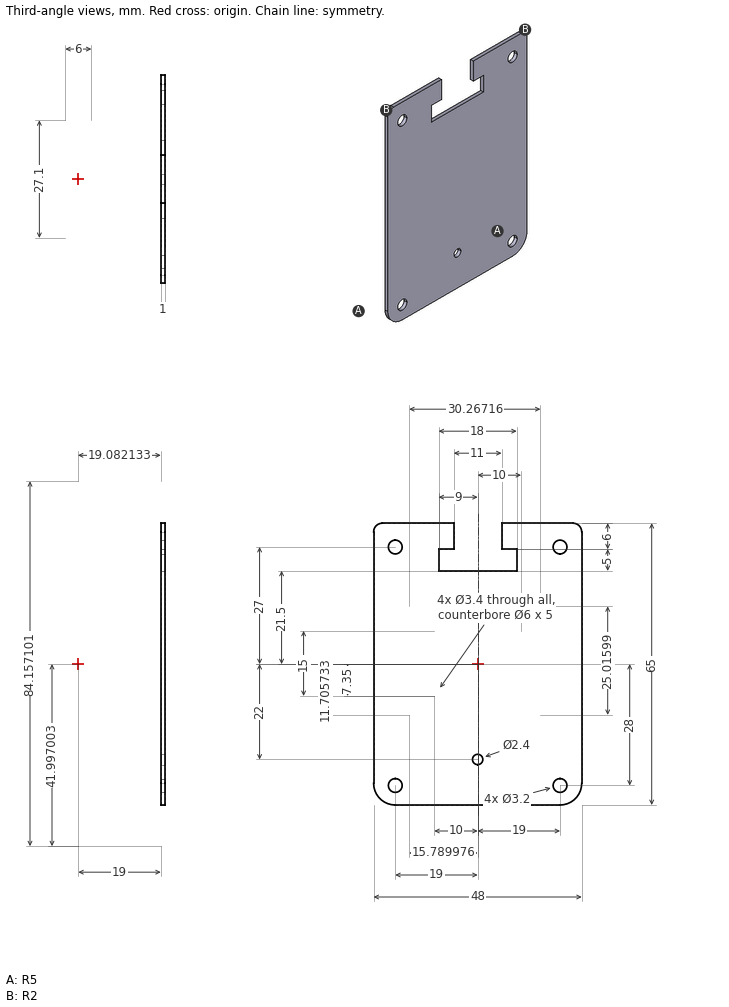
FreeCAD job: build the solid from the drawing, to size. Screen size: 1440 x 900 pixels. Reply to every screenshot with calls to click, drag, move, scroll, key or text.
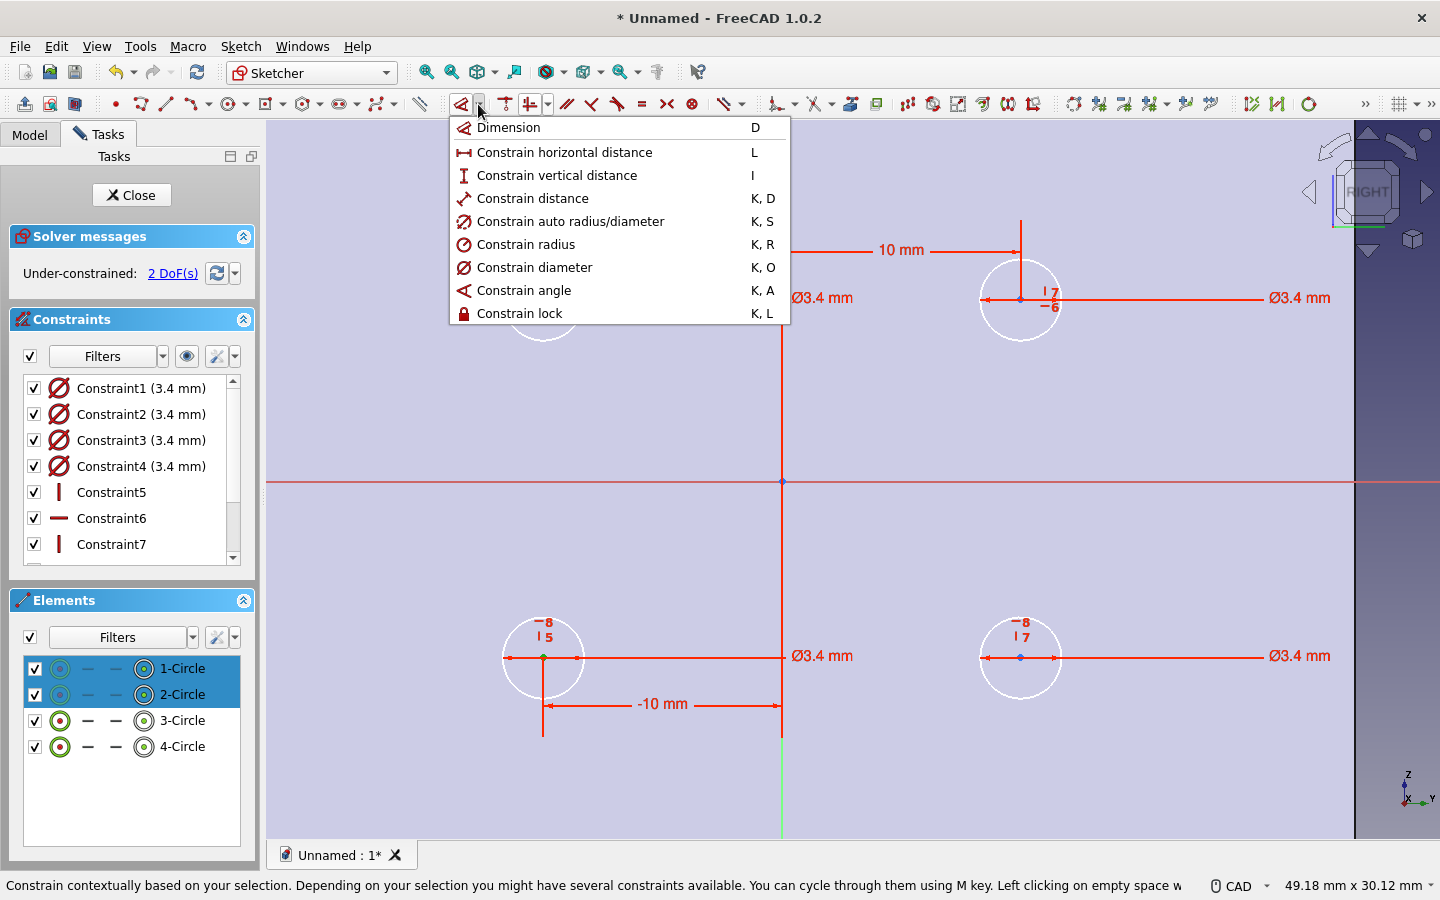
click(620, 176)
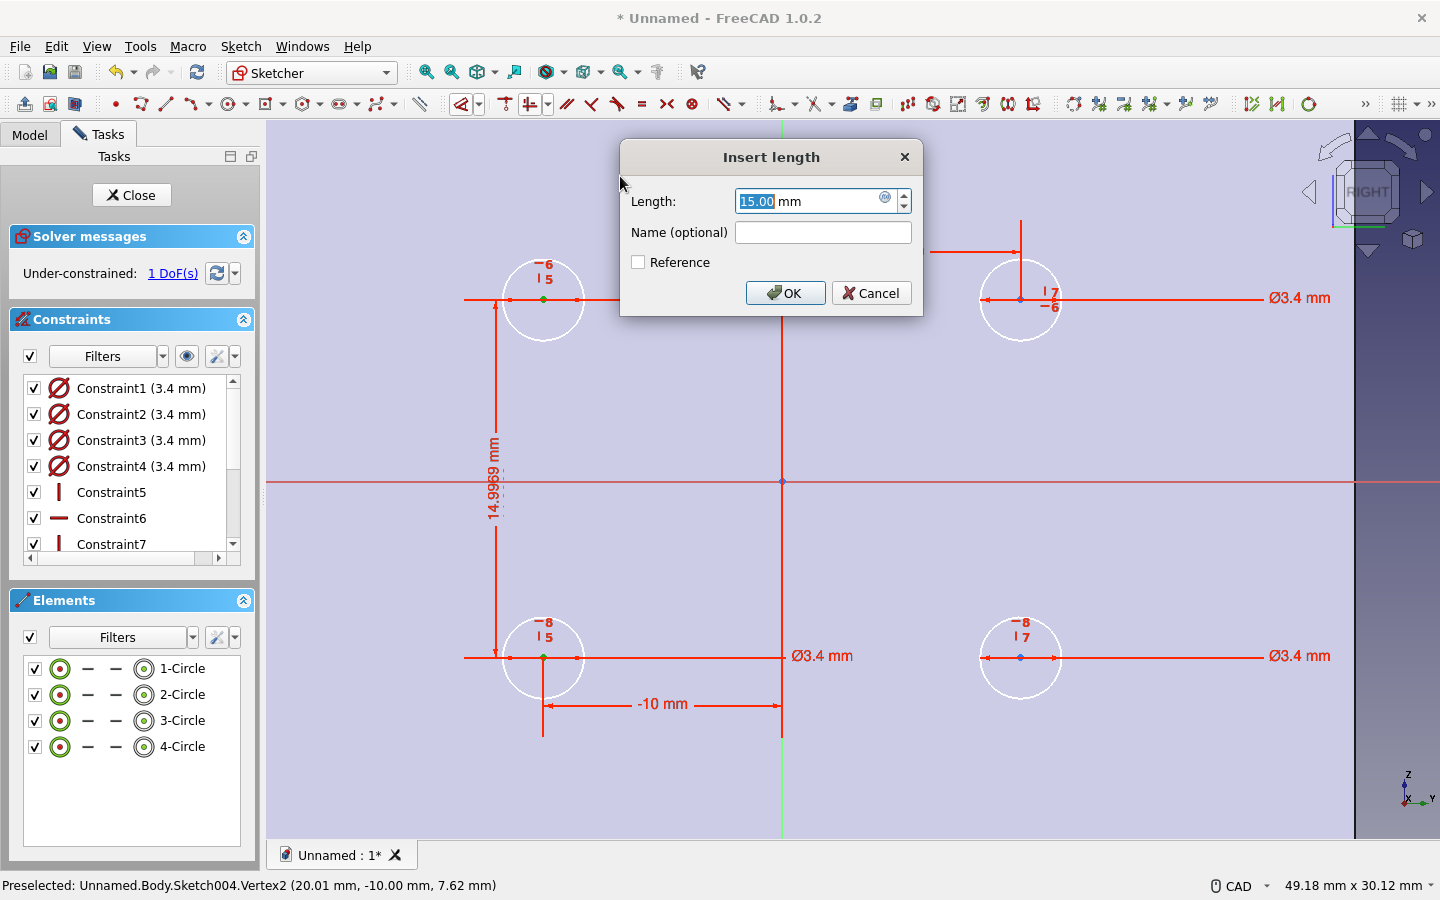
text(15)
key(Return)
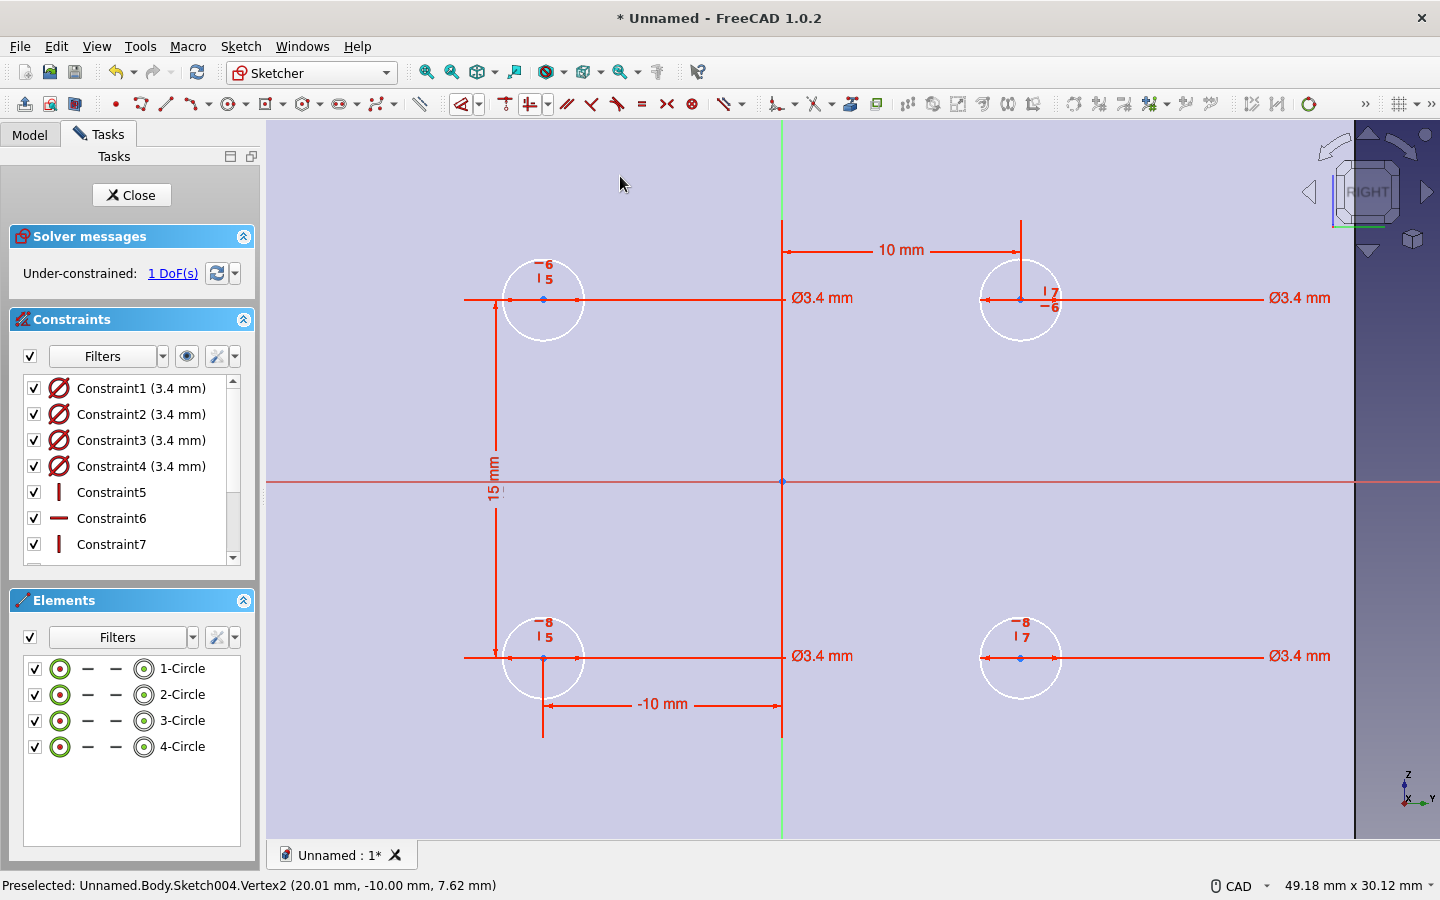
click(543, 658)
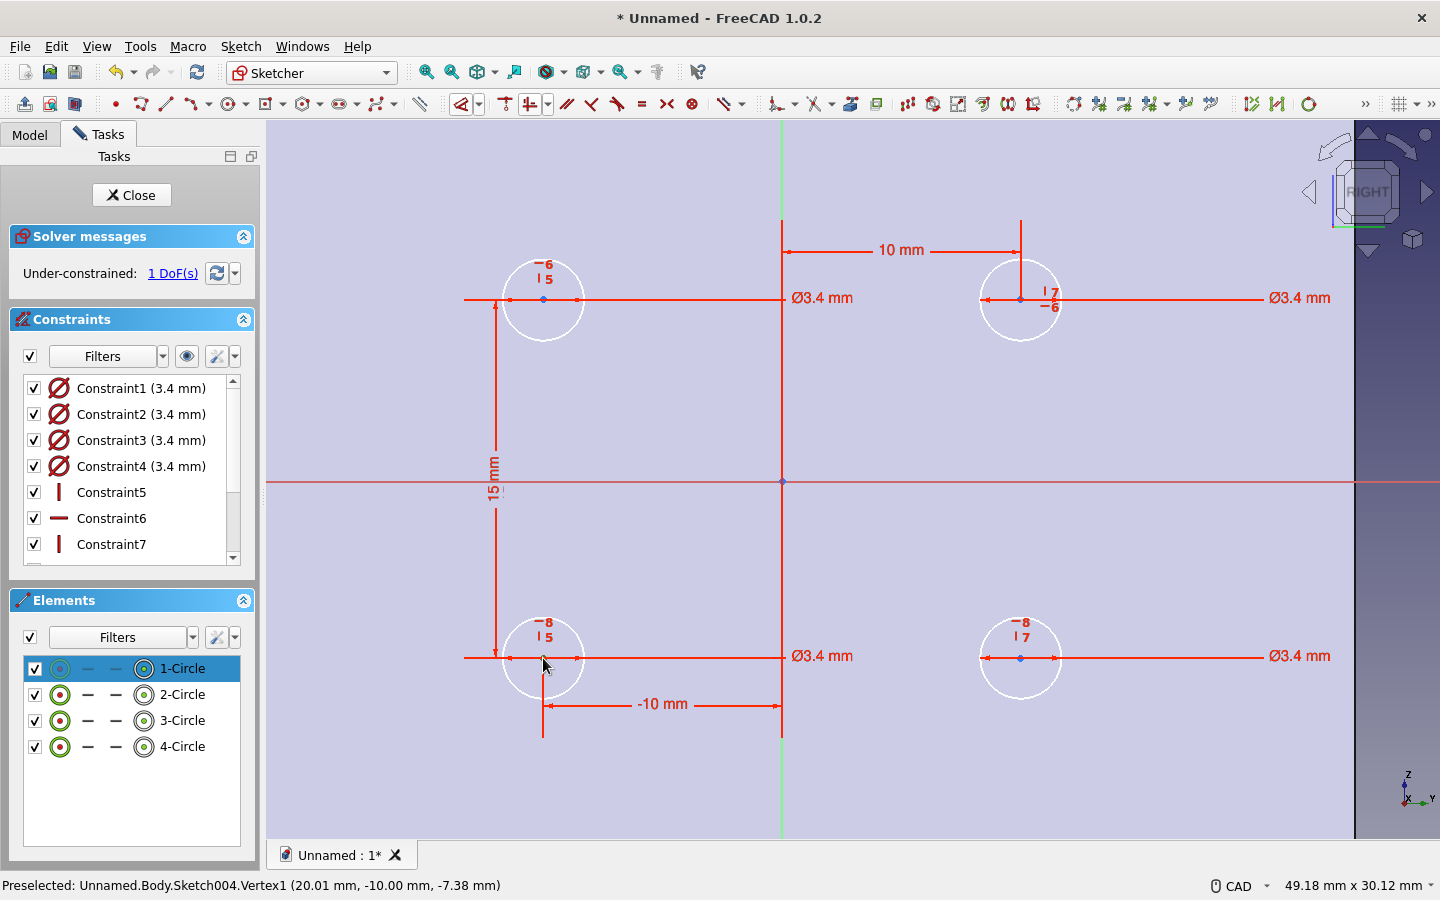
key(i)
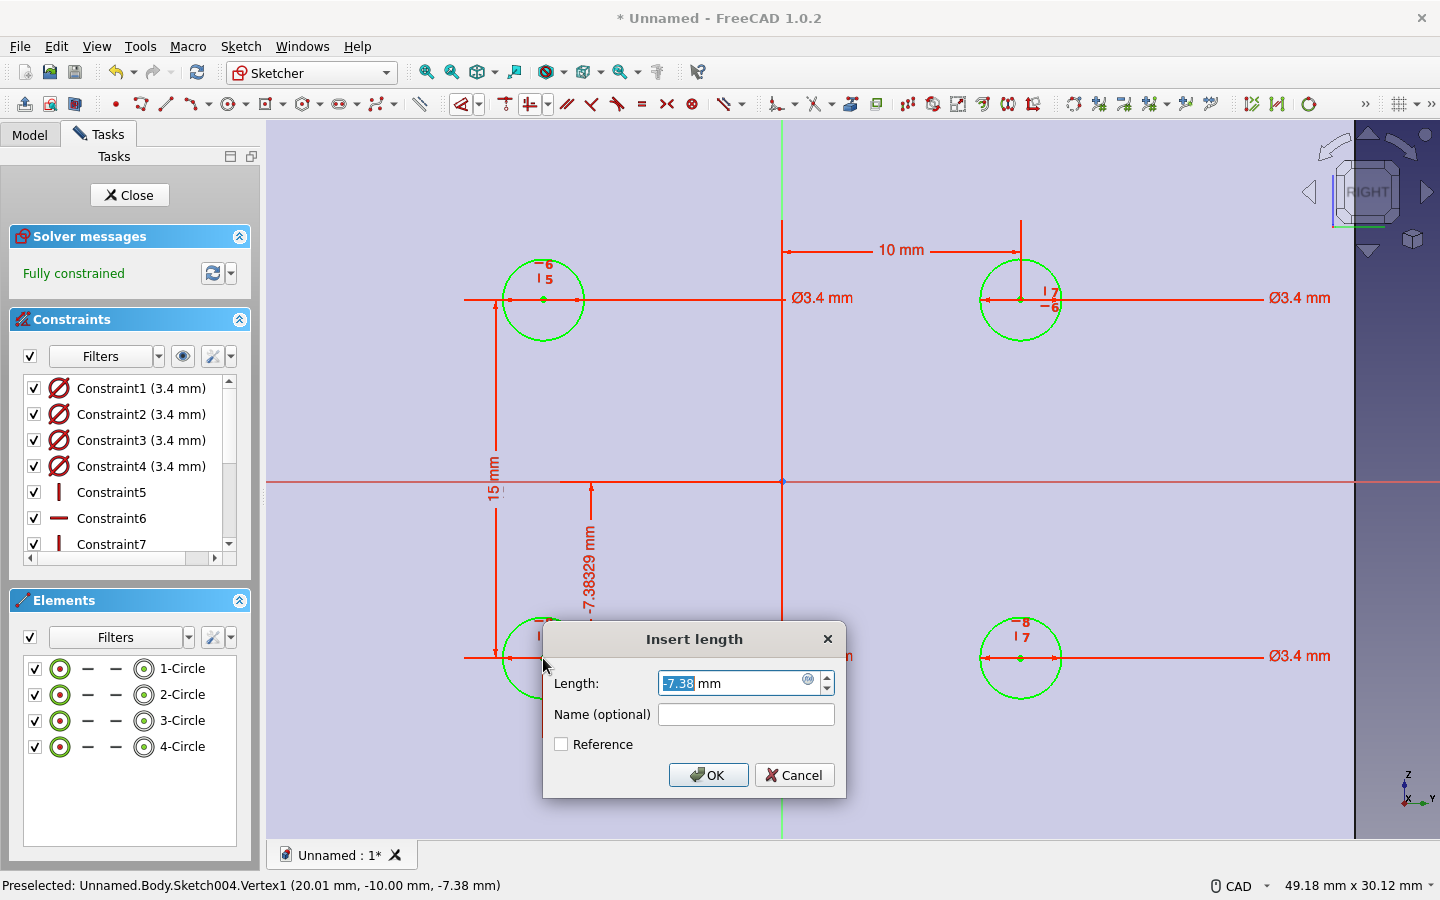
text(-7.35)
key(Return)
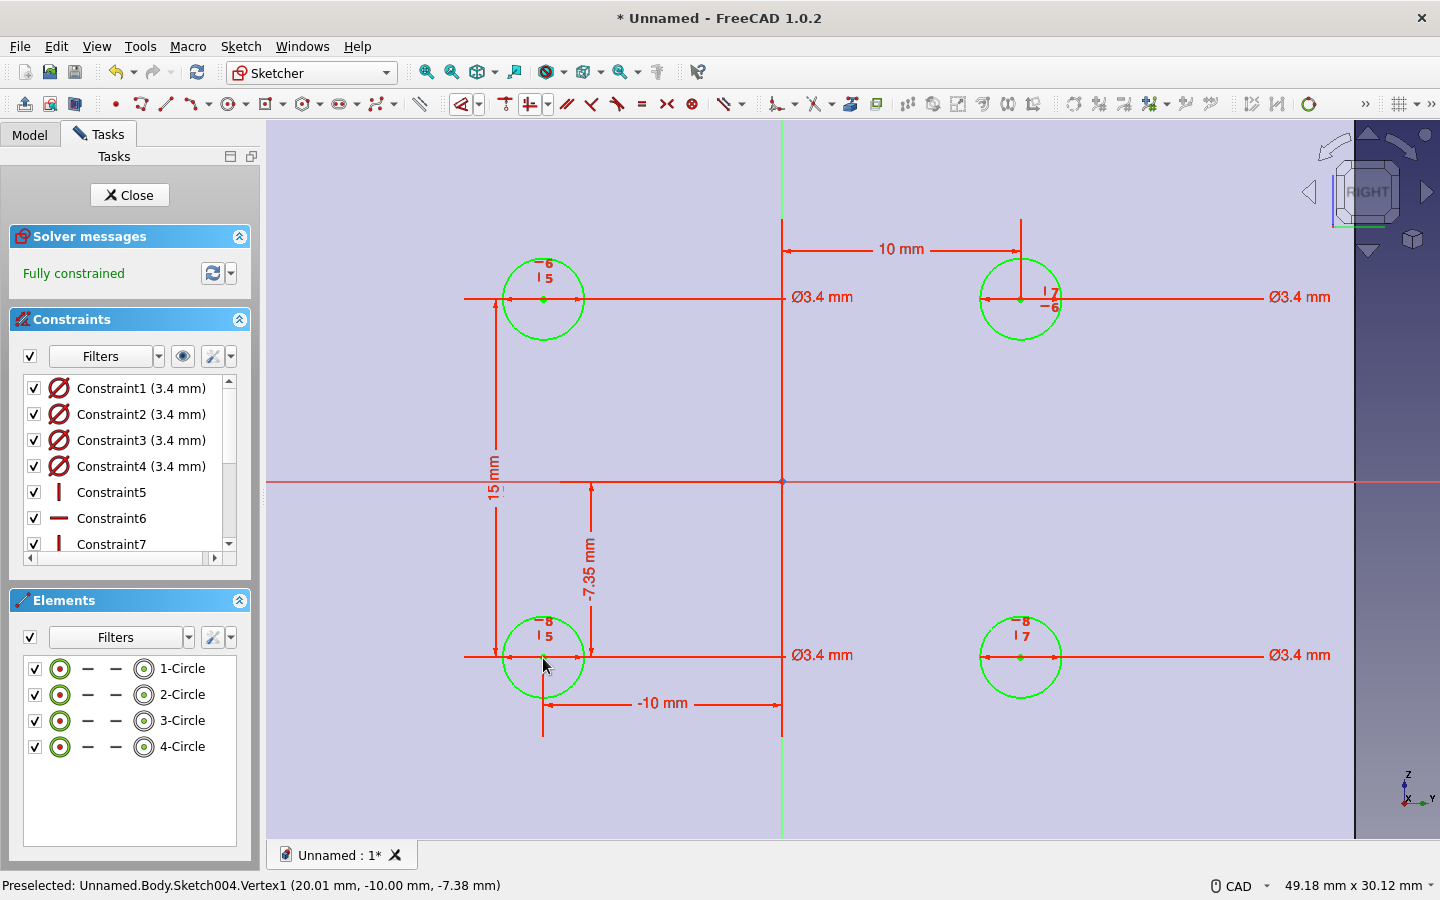
click(130, 195)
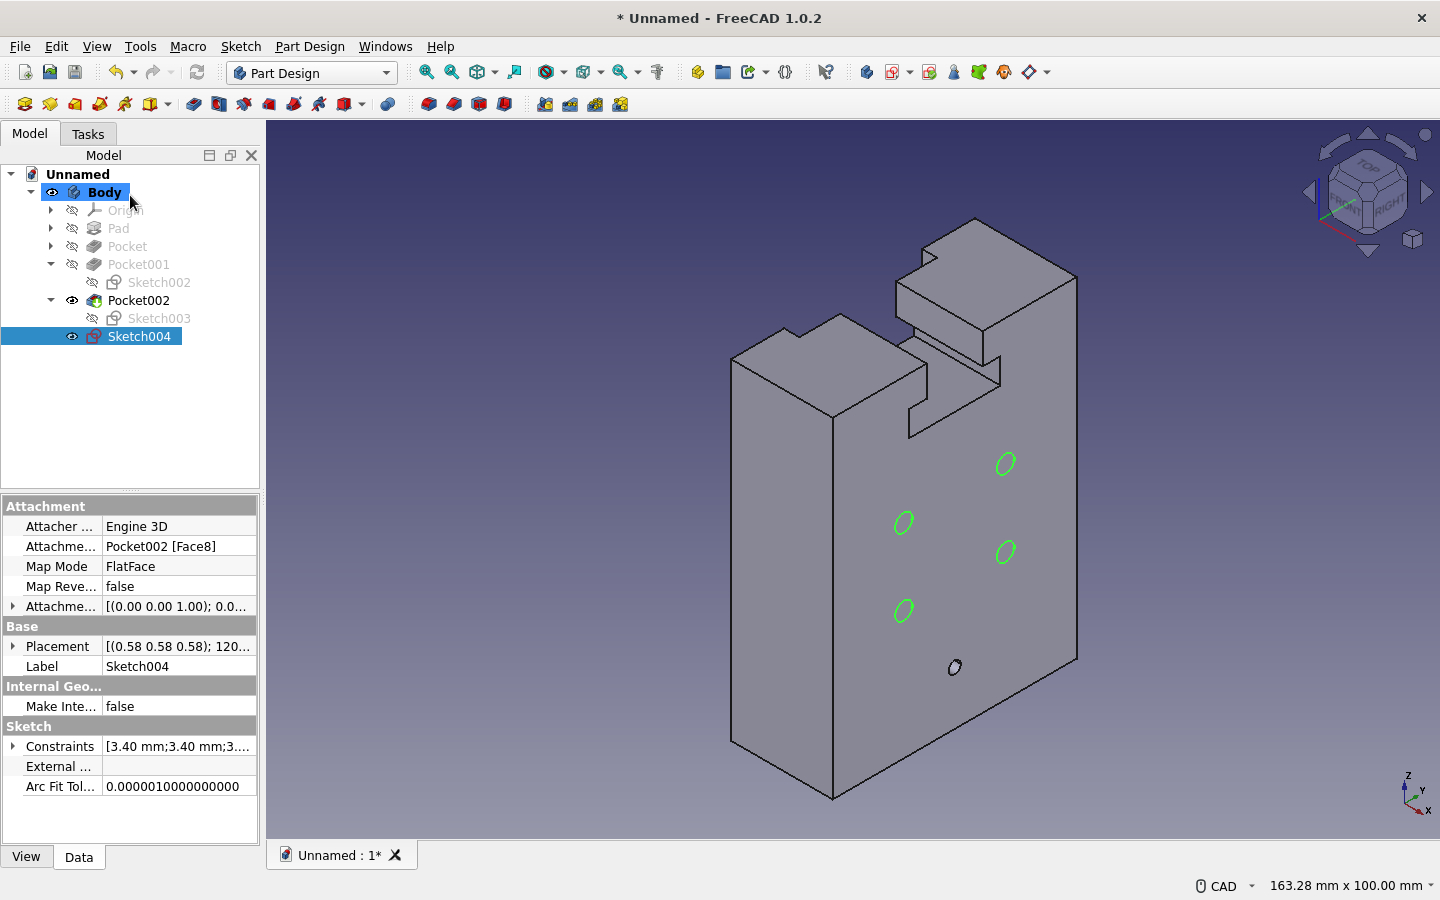
click(219, 104)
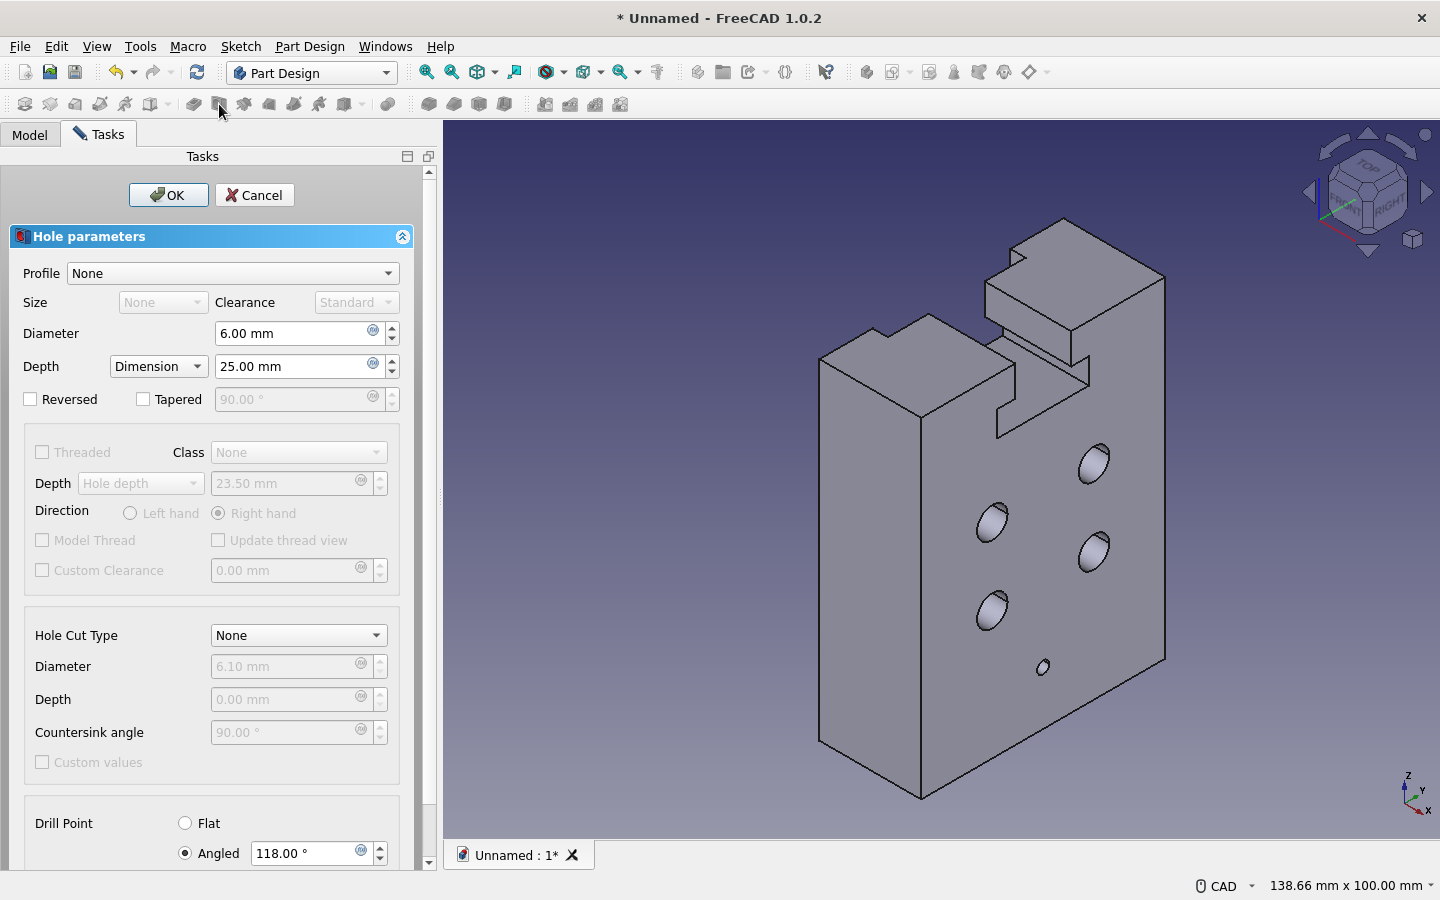
triple_click(300, 334)